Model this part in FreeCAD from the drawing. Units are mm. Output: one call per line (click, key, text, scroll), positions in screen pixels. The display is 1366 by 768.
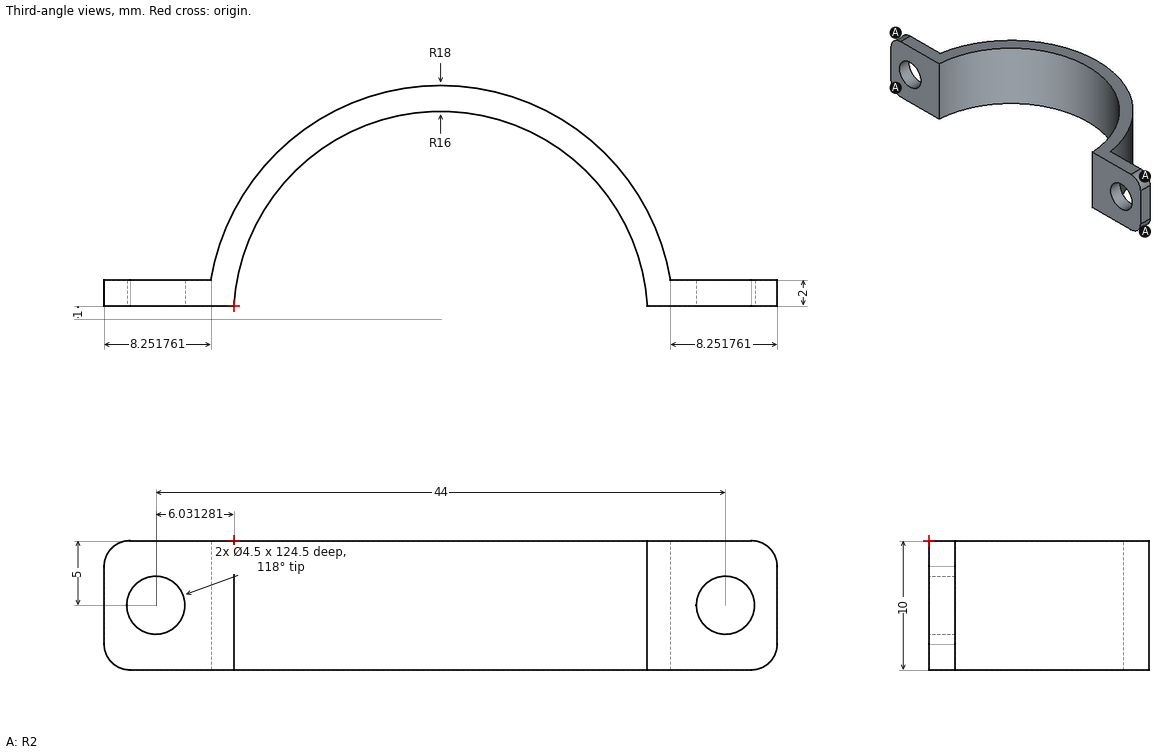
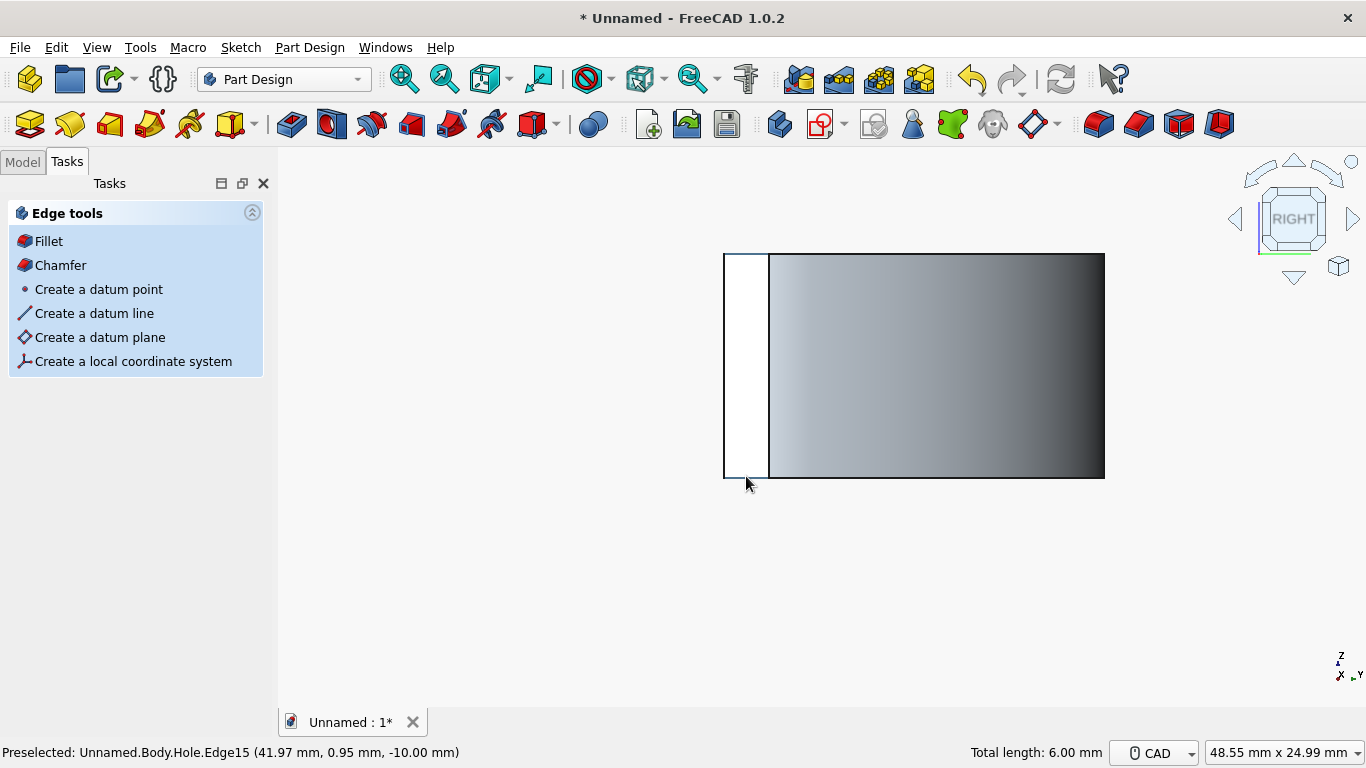
click(406, 80)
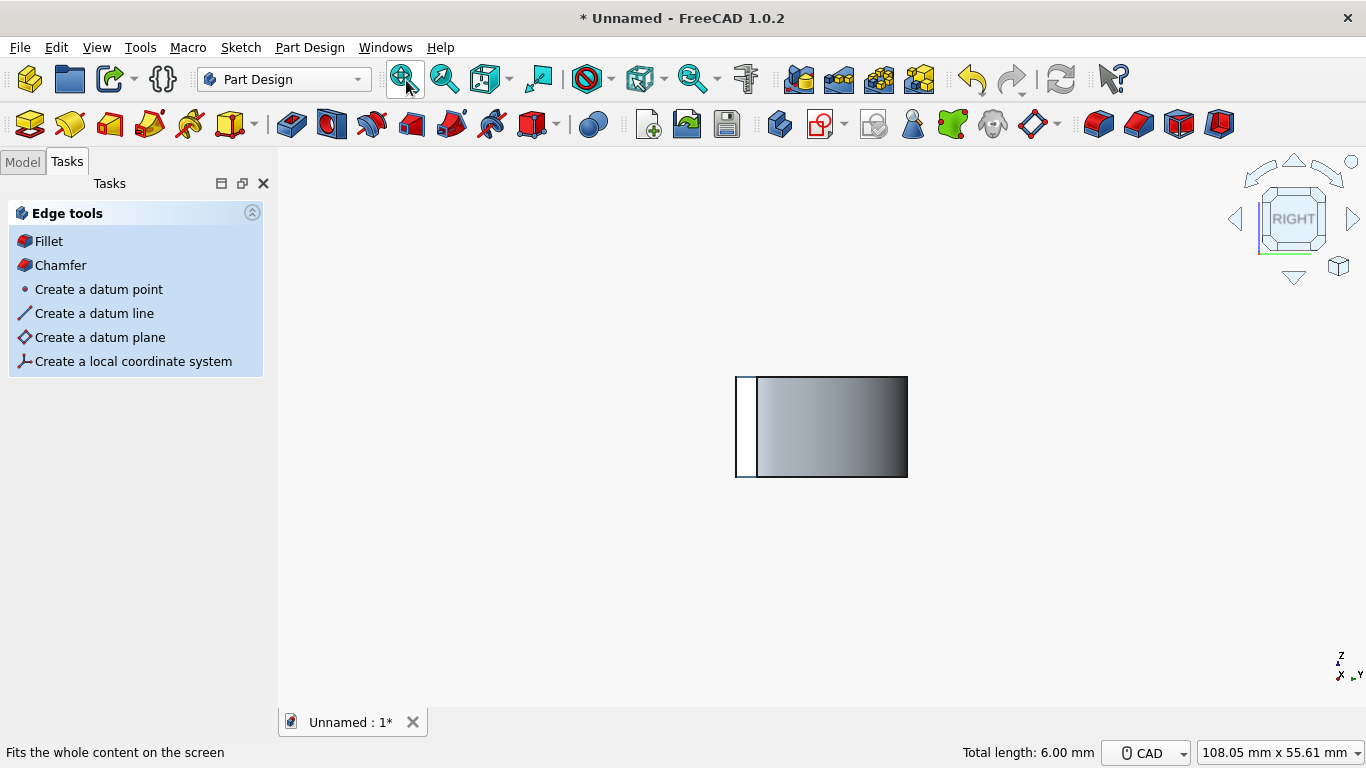
key(5)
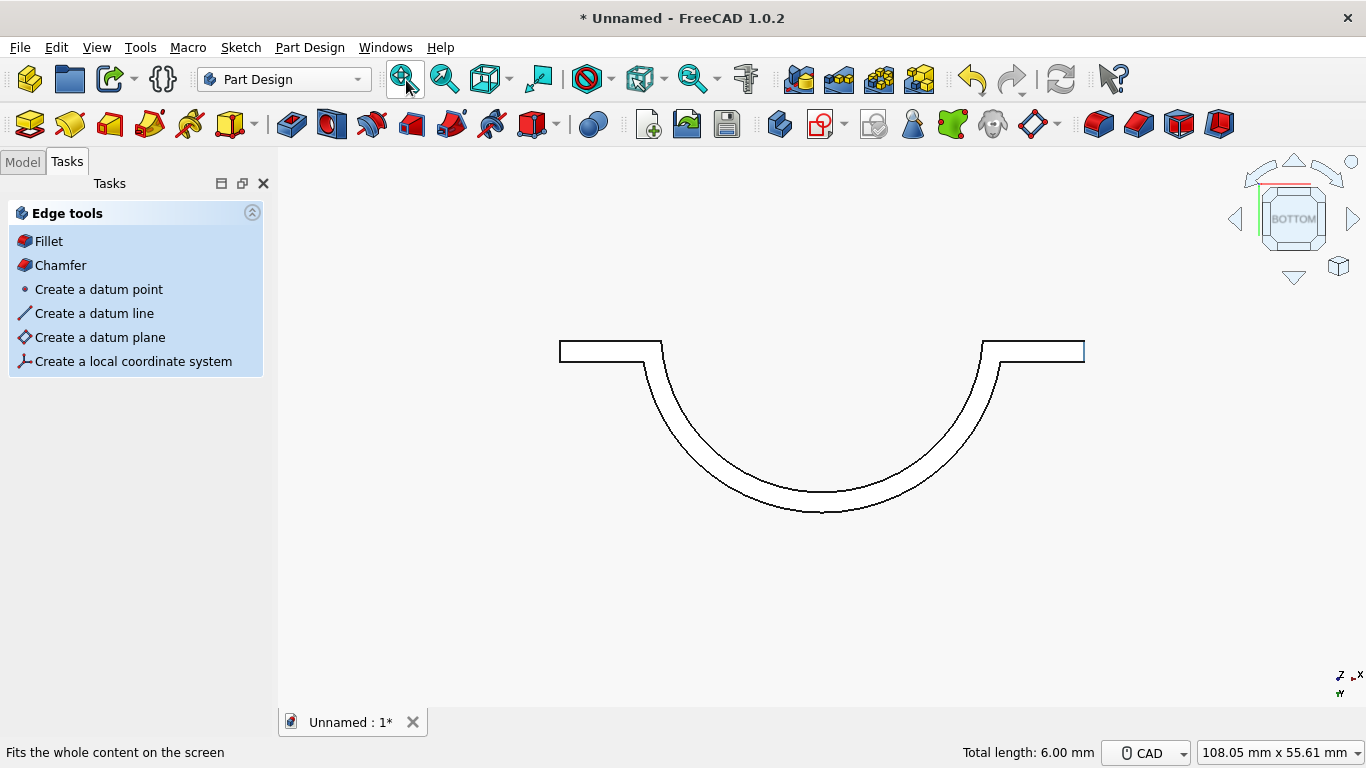
click(560, 350, ctrl)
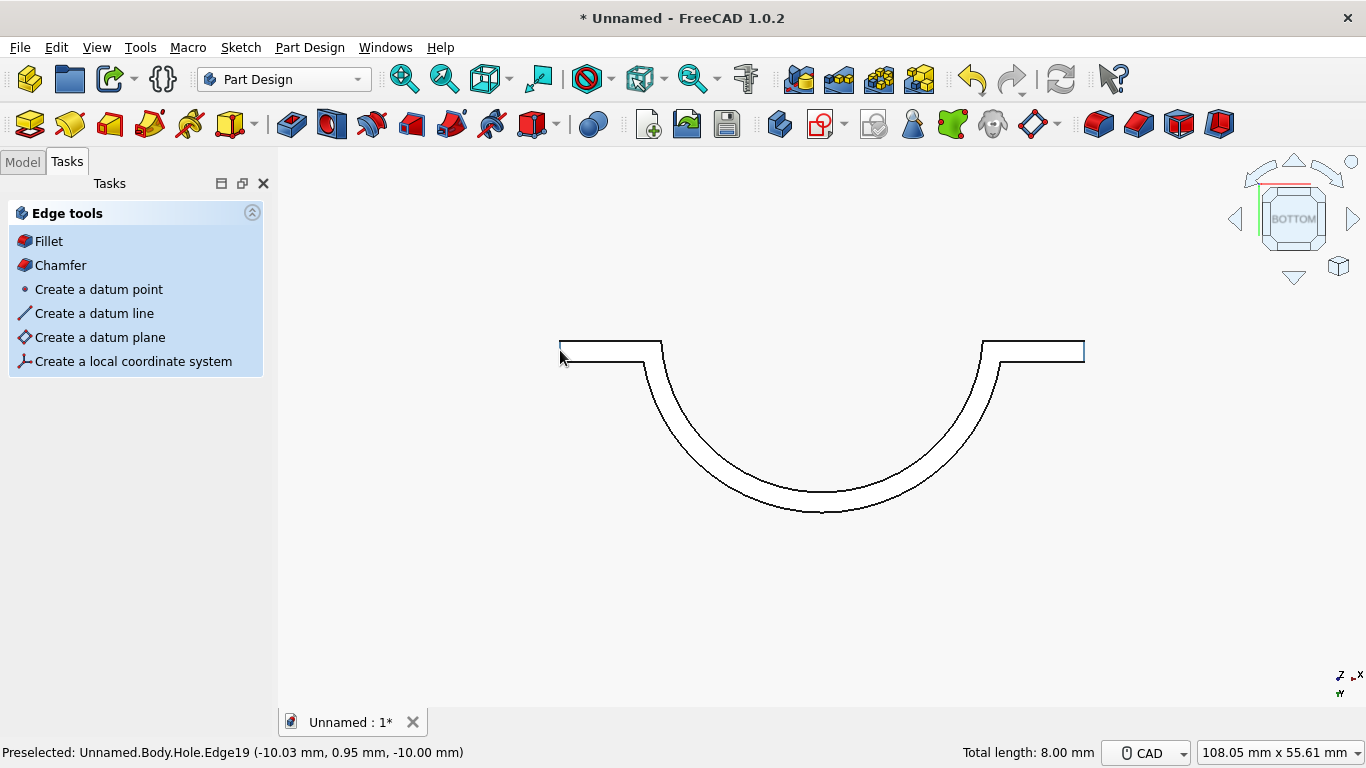
click(1100, 124)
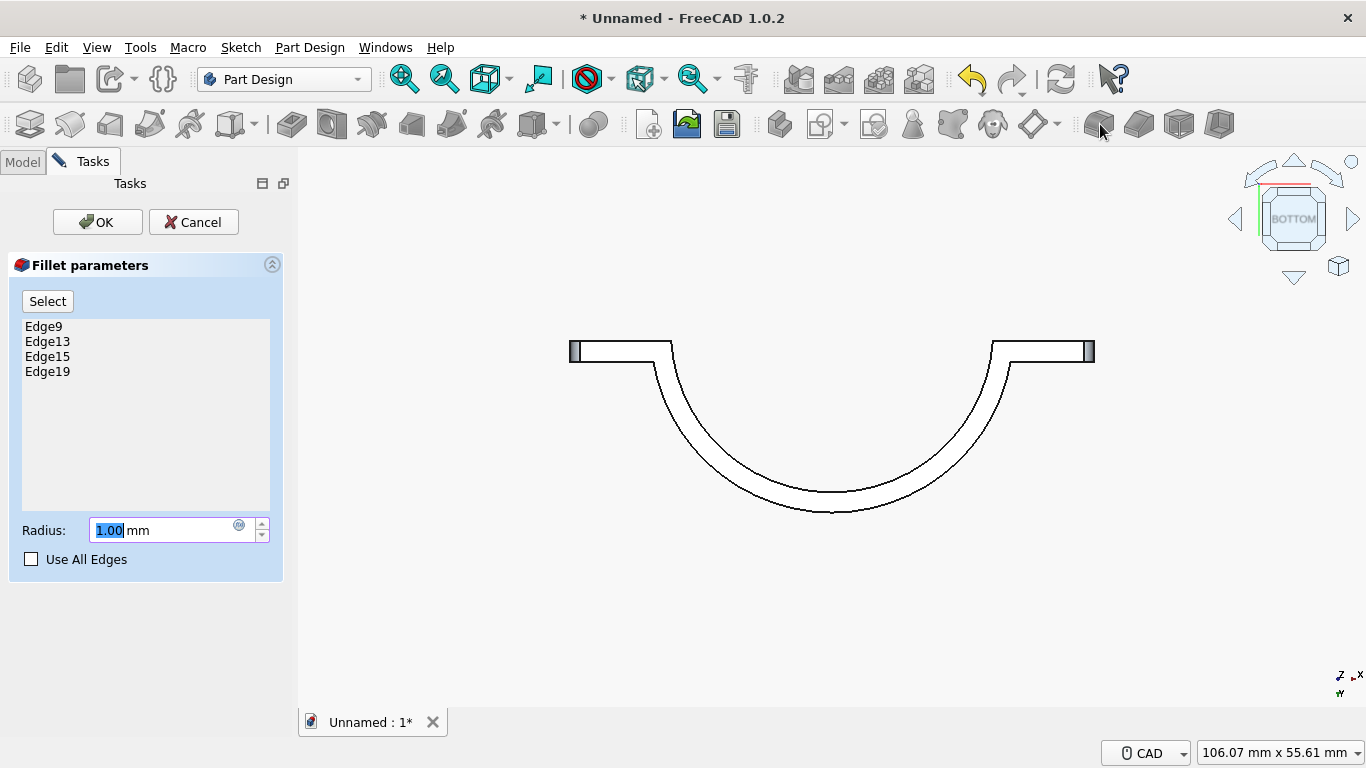
text(2)
key(Tab)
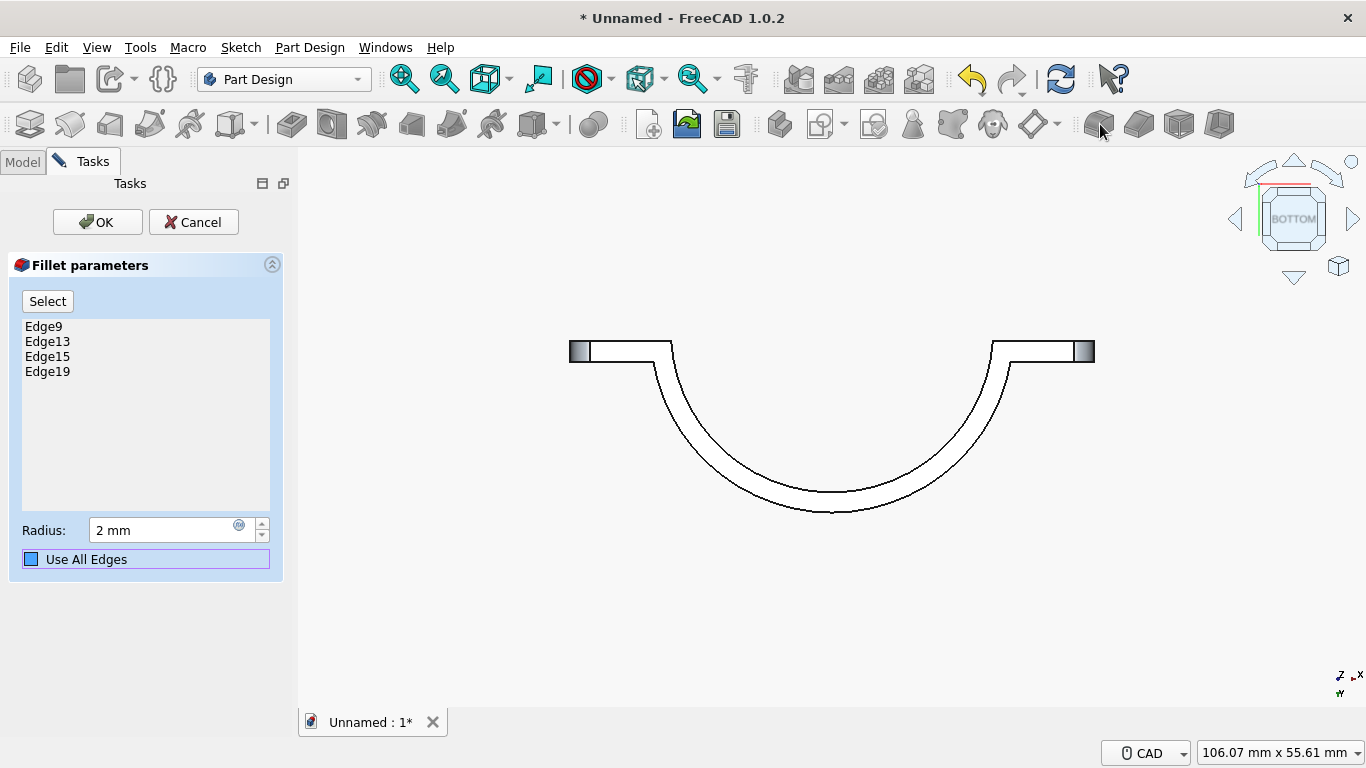
click(98, 222)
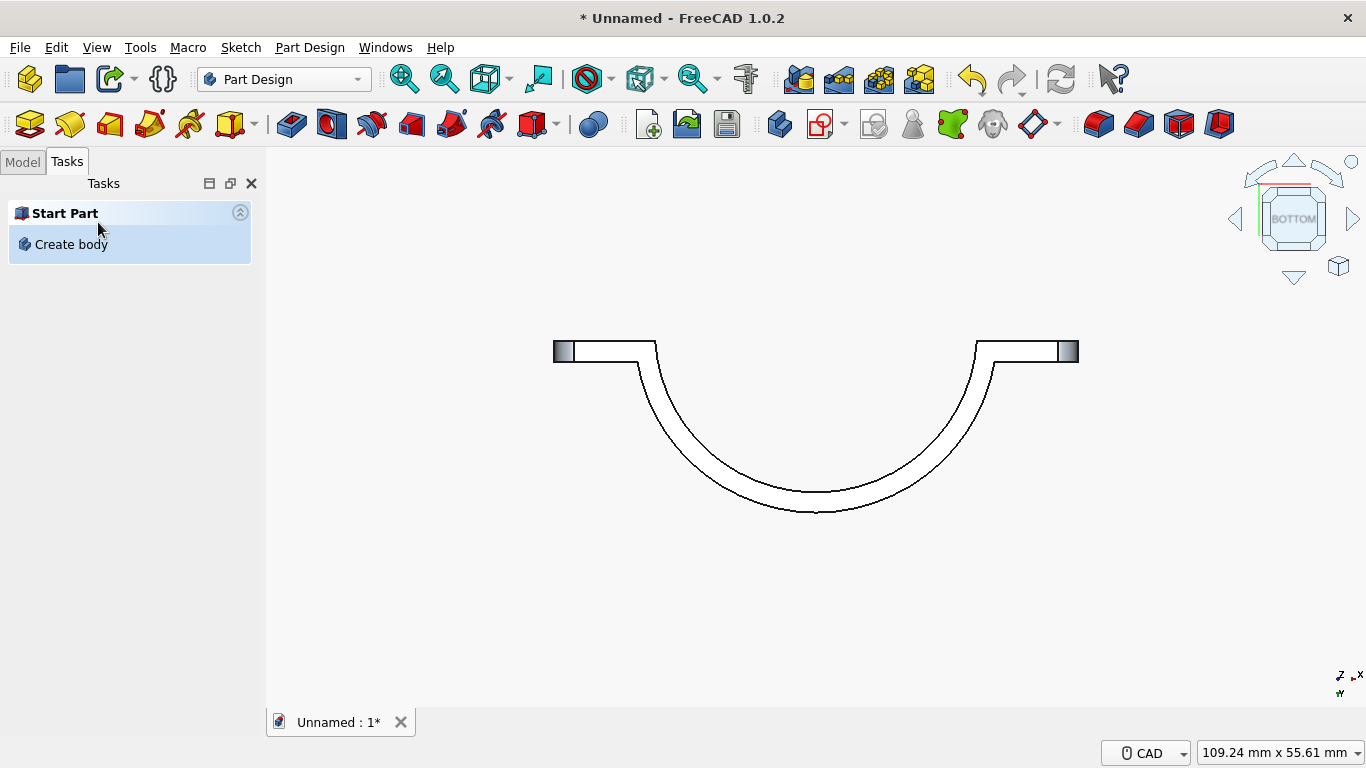
key(0)